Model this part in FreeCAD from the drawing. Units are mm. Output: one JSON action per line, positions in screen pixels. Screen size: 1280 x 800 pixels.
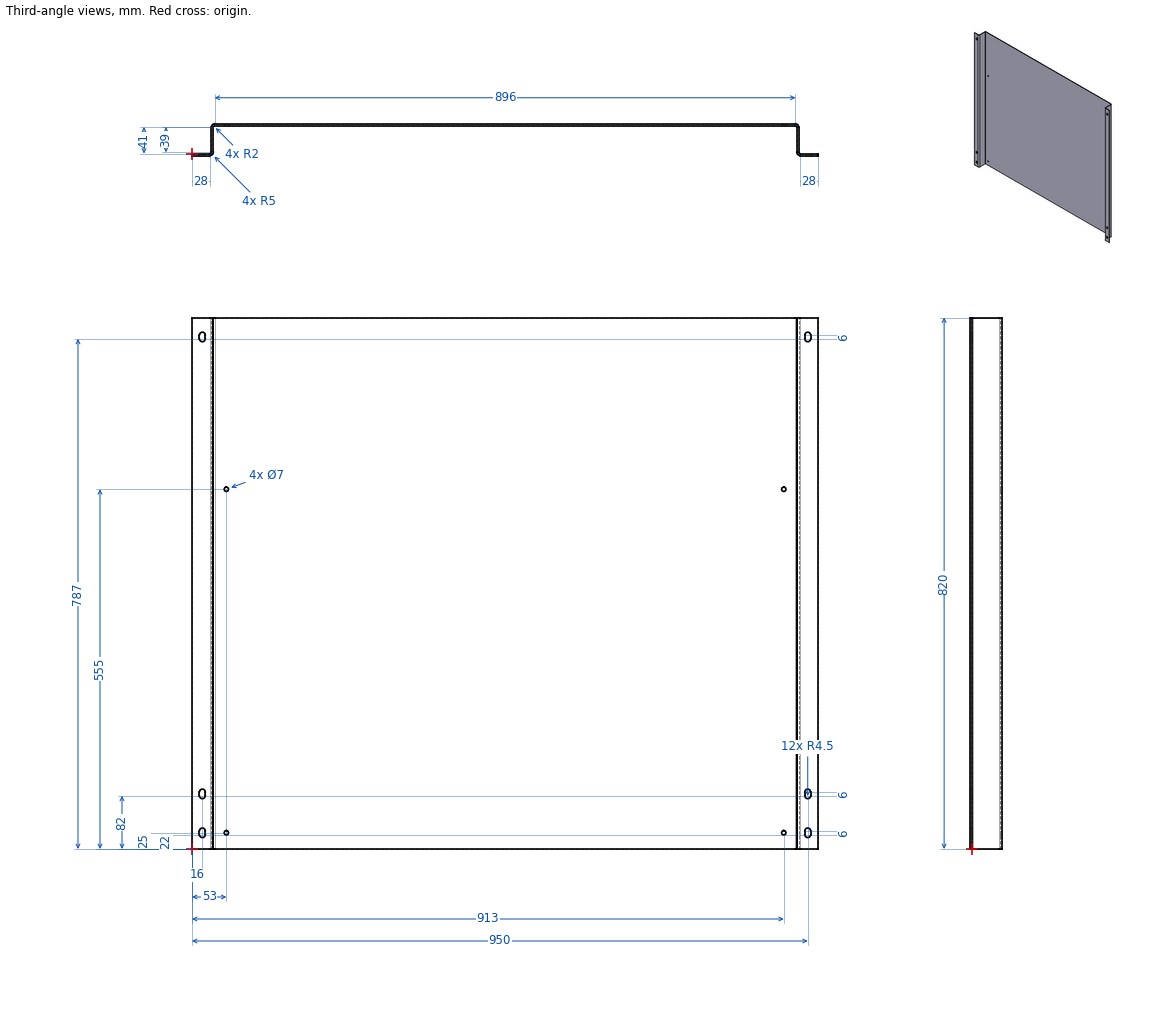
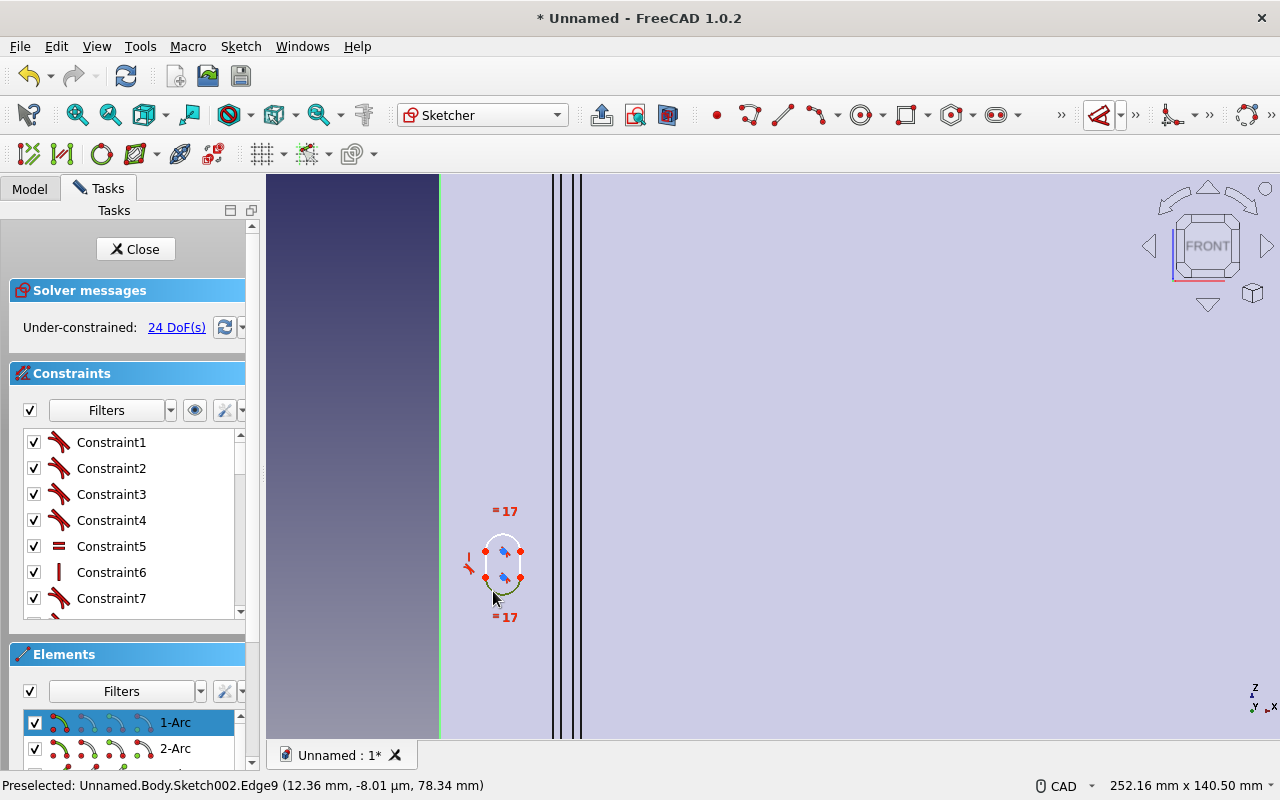
{"action": "scroll", "coordinate": [498, 601], "scroll_direction": "down", "scroll_amount": 11}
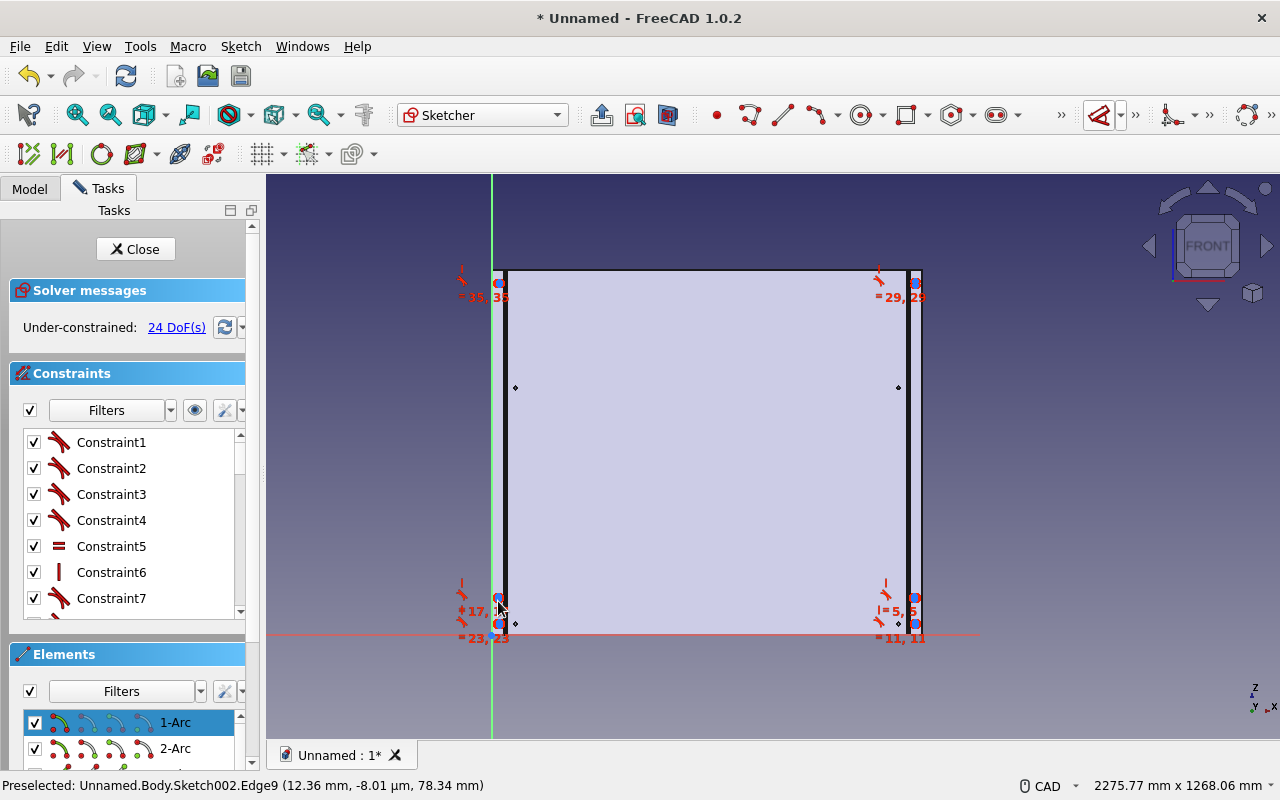
{"action": "scroll", "coordinate": [498, 627], "scroll_direction": "up", "scroll_amount": 10}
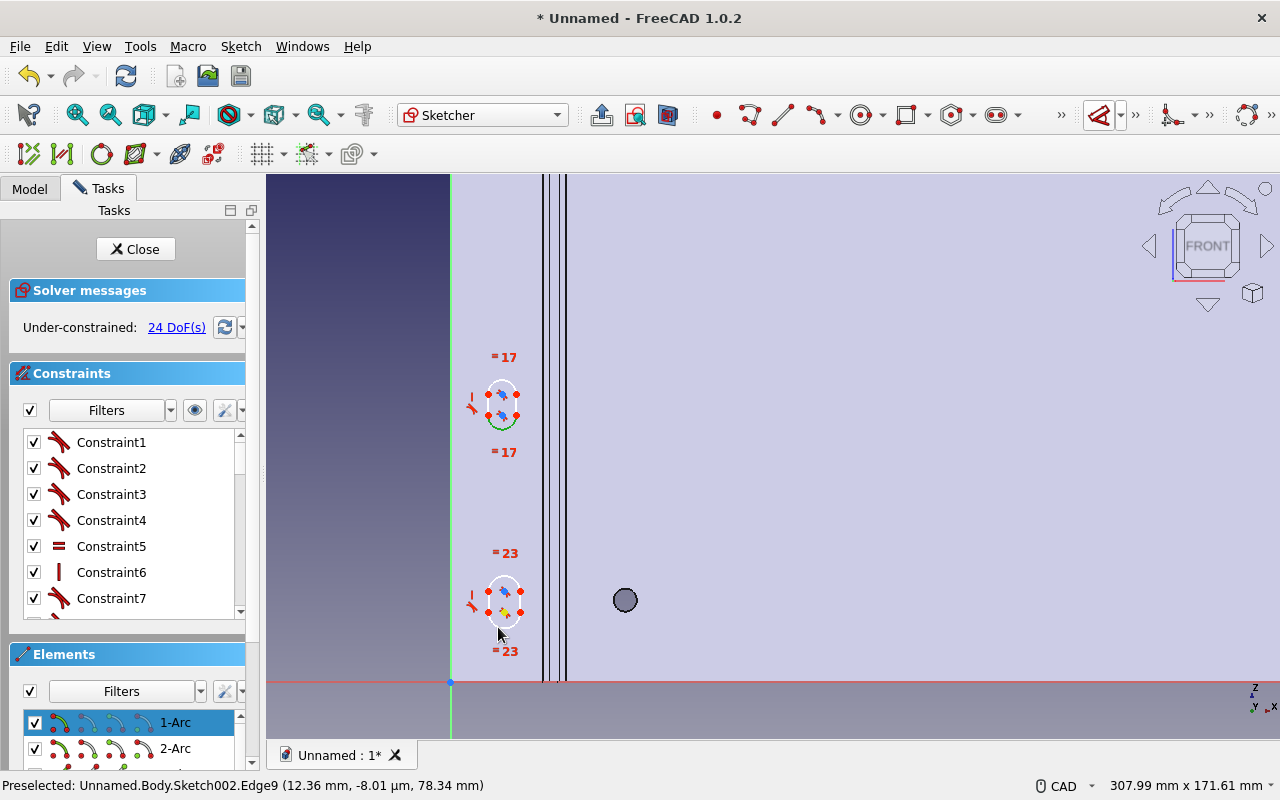
{"action": "left_click", "coordinate": [495, 625]}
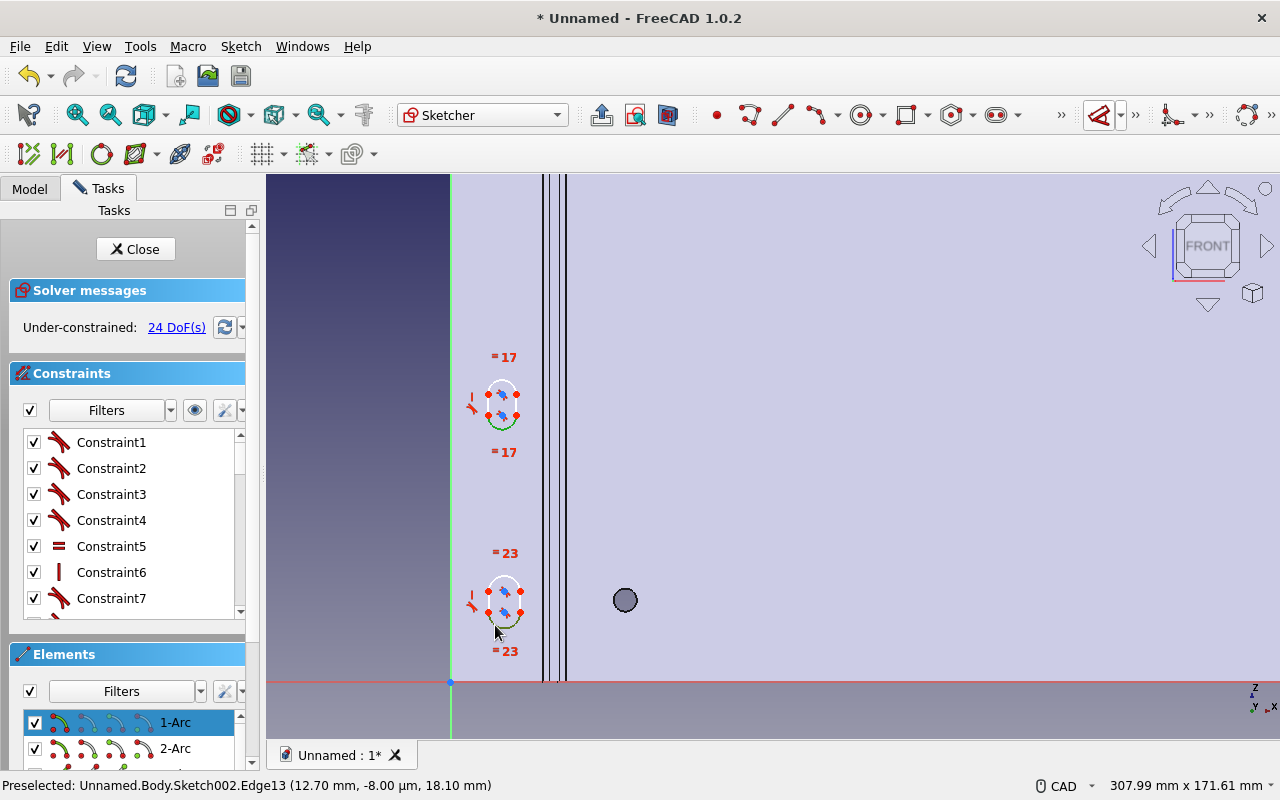
{"action": "scroll", "coordinate": [498, 627], "scroll_direction": "down", "scroll_amount": 10}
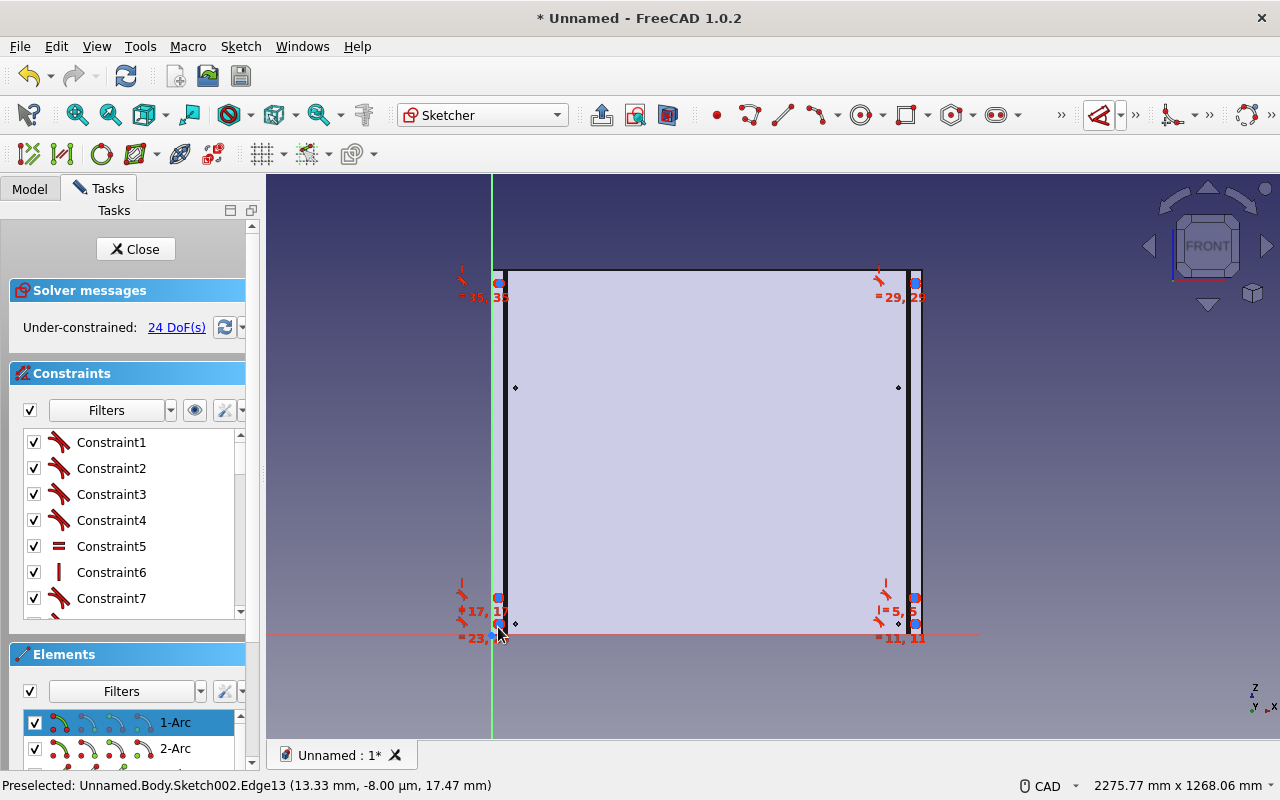
{"action": "scroll", "coordinate": [914, 287], "scroll_direction": "up", "scroll_amount": 11}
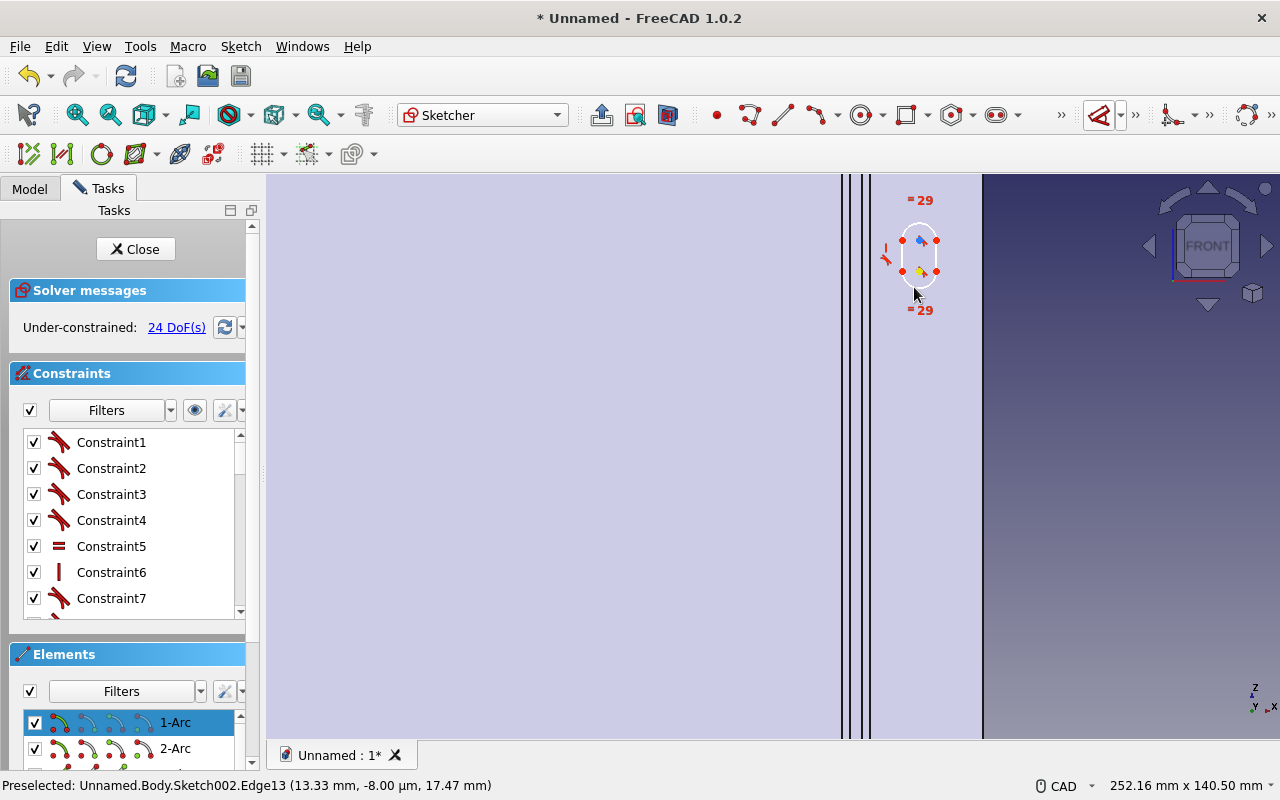
{"action": "left_click", "coordinate": [909, 285]}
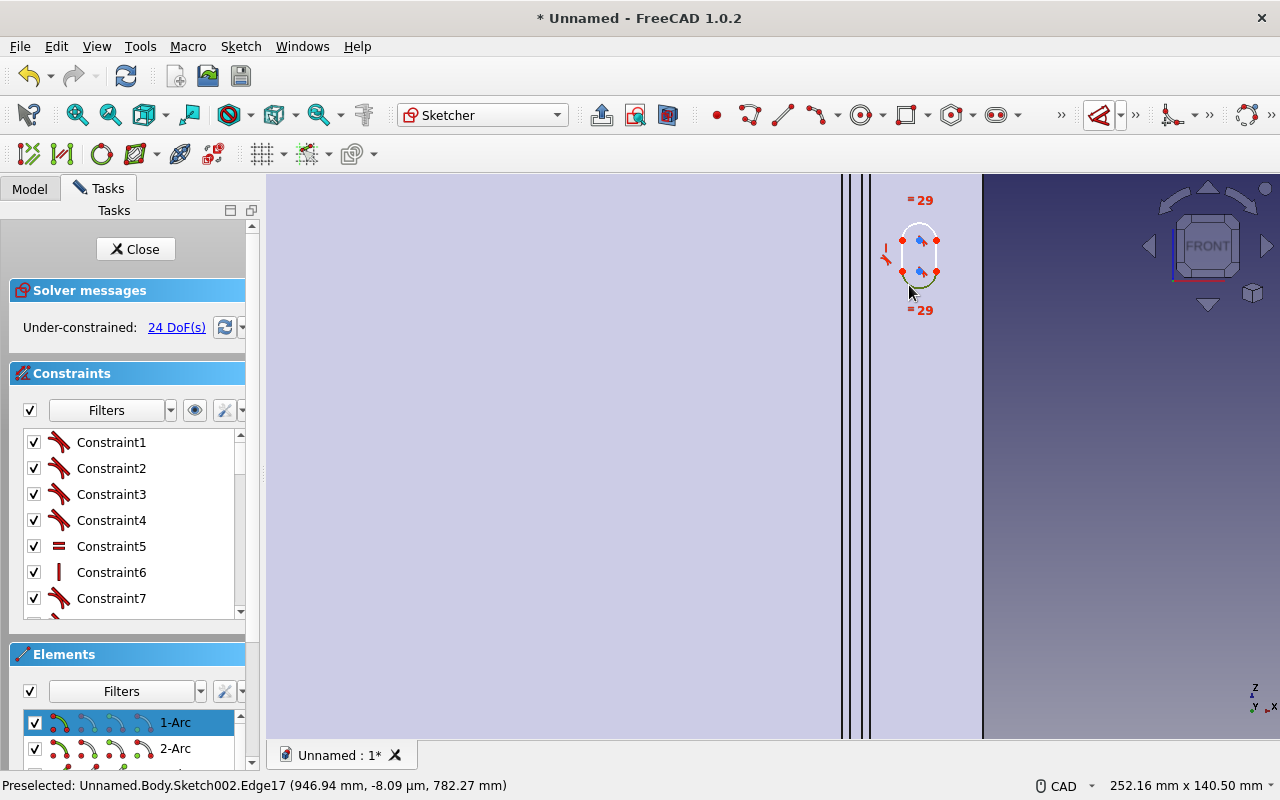
{"action": "scroll", "coordinate": [915, 286], "scroll_direction": "down", "scroll_amount": 11}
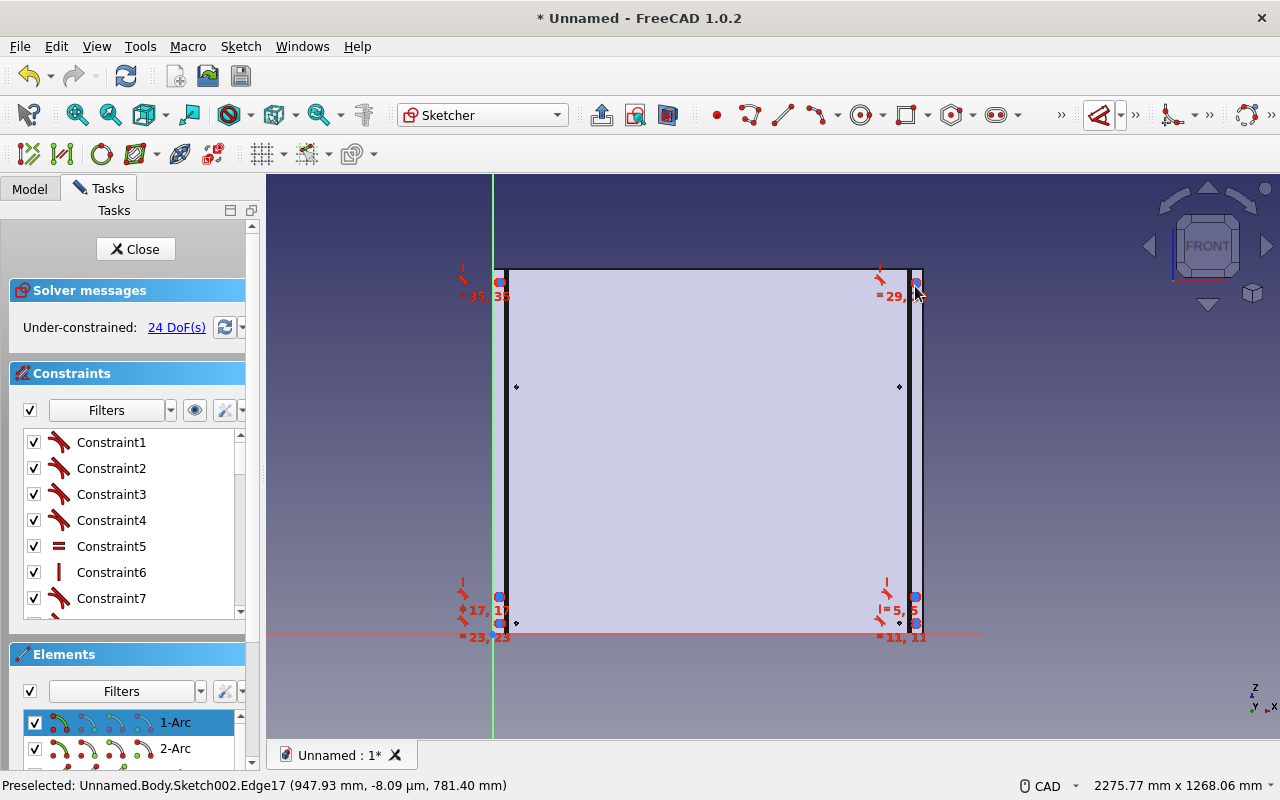
{"action": "scroll", "coordinate": [499, 286], "scroll_direction": "up", "scroll_amount": 10}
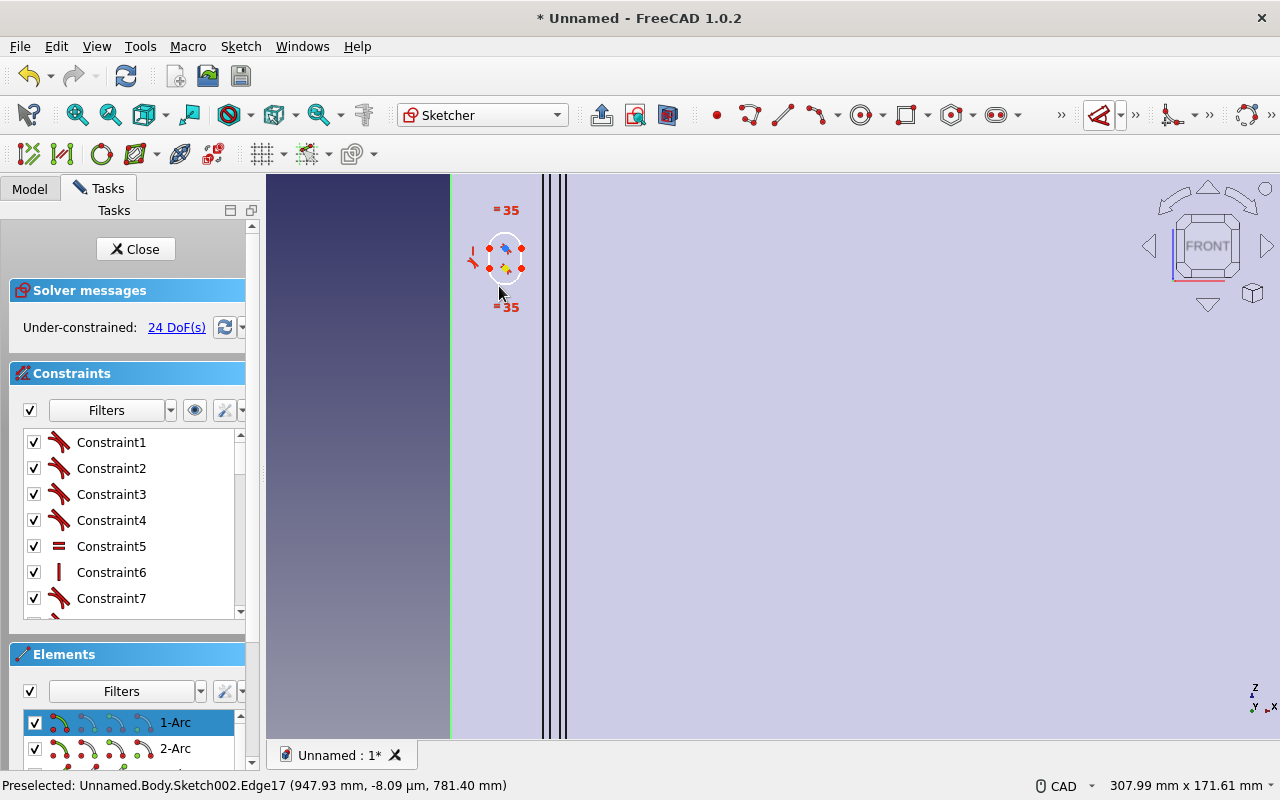
{"action": "left_click", "coordinate": [496, 281]}